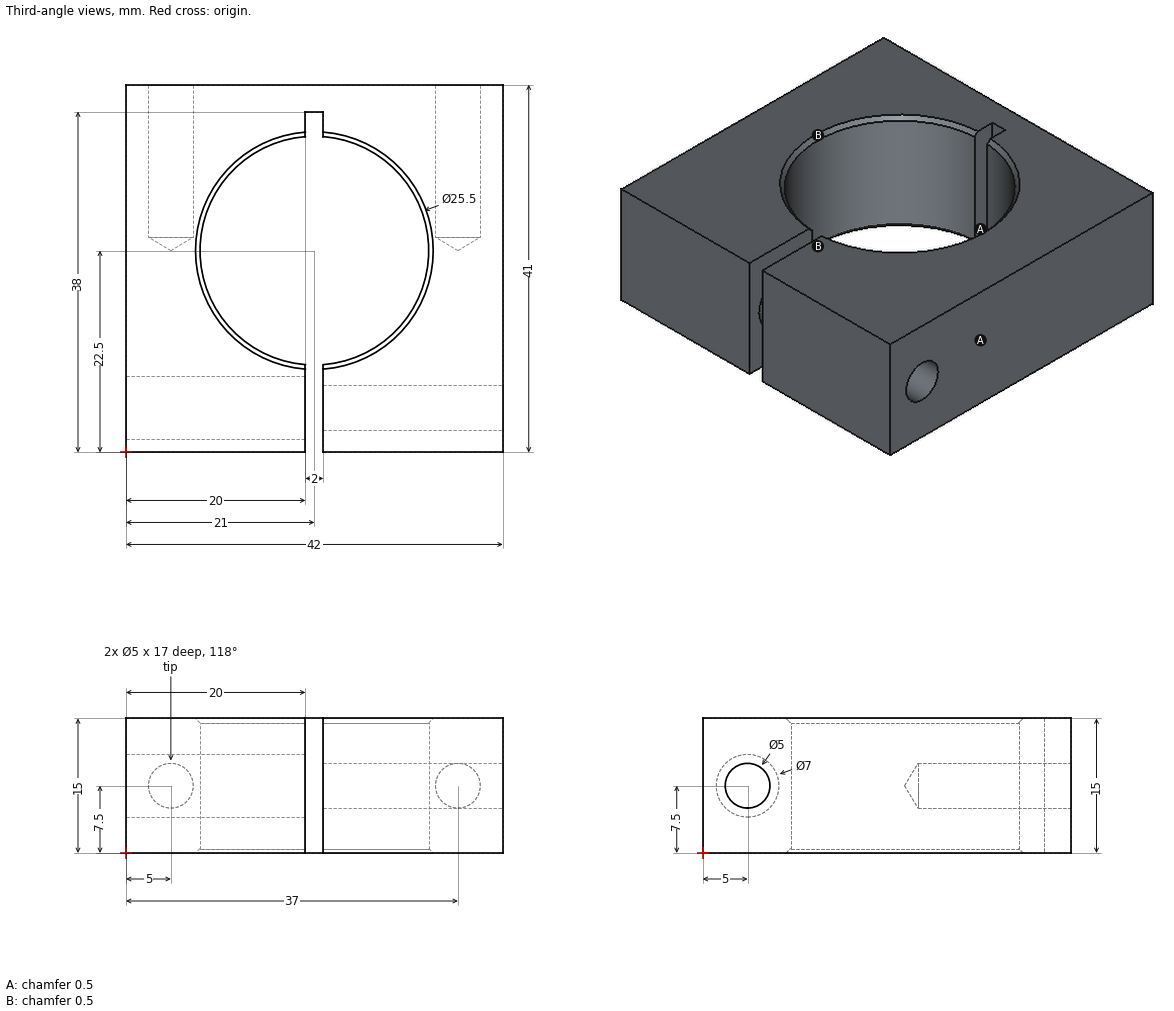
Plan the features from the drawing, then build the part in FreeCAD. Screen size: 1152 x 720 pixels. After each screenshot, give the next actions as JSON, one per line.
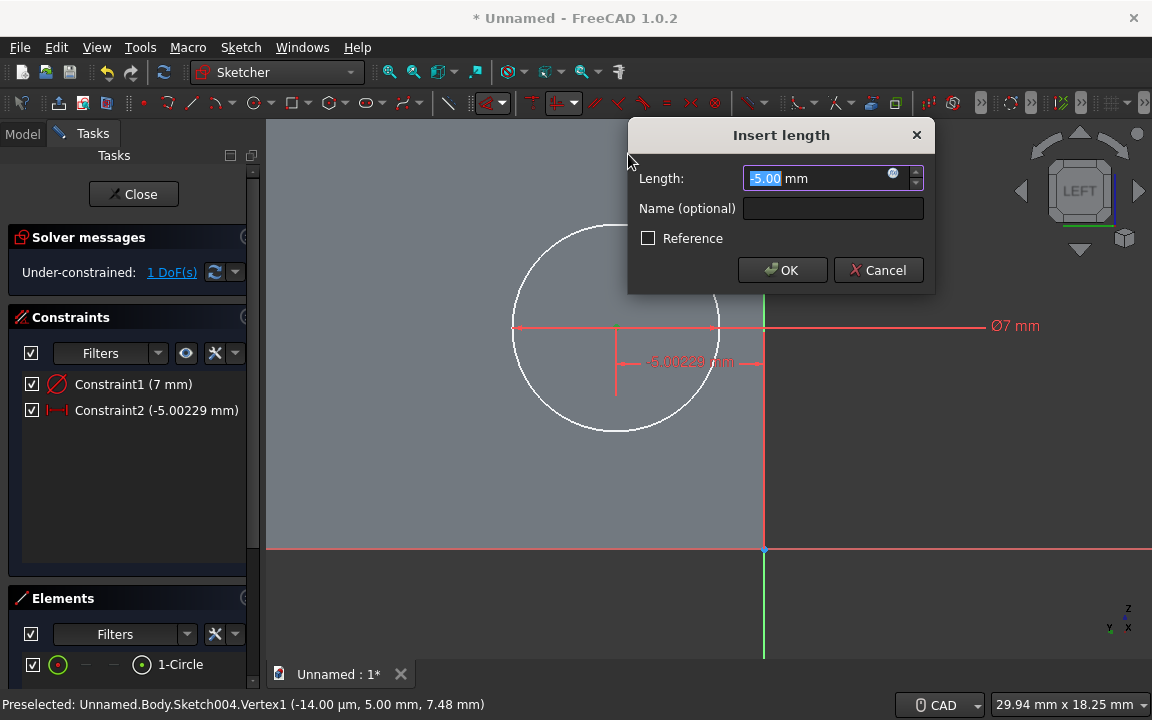
{"action": "type", "text": "-5"}
{"action": "key", "text": "Return"}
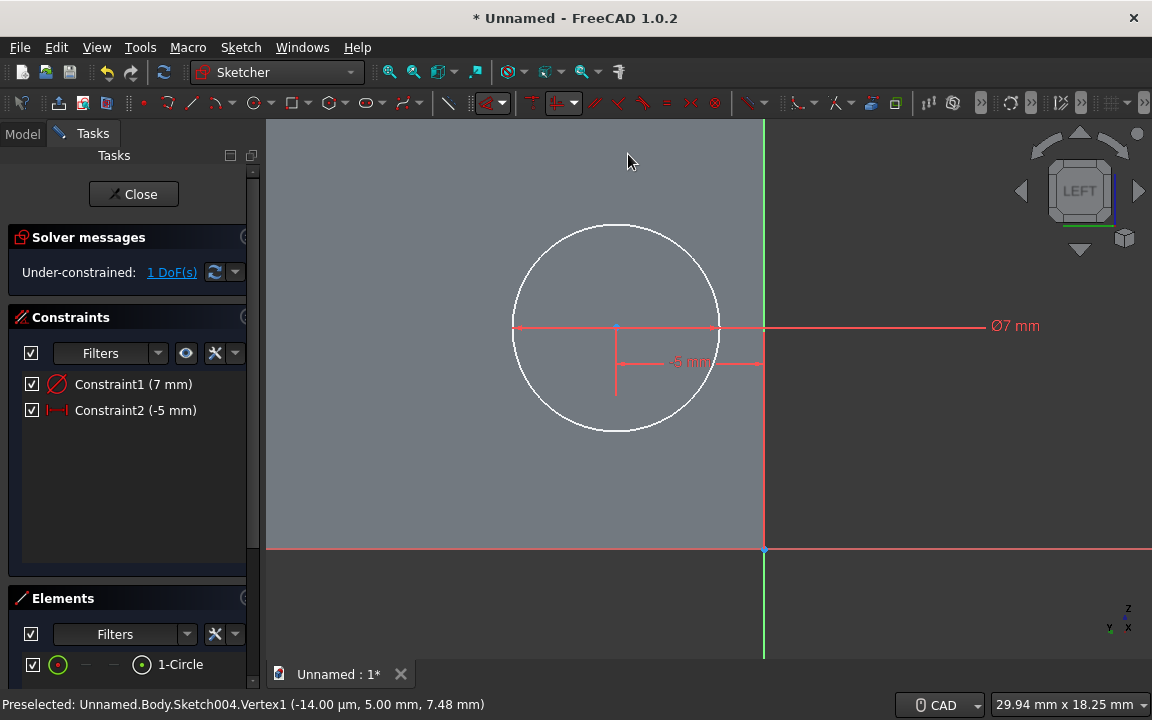
{"action": "left_click", "coordinate": [616, 328]}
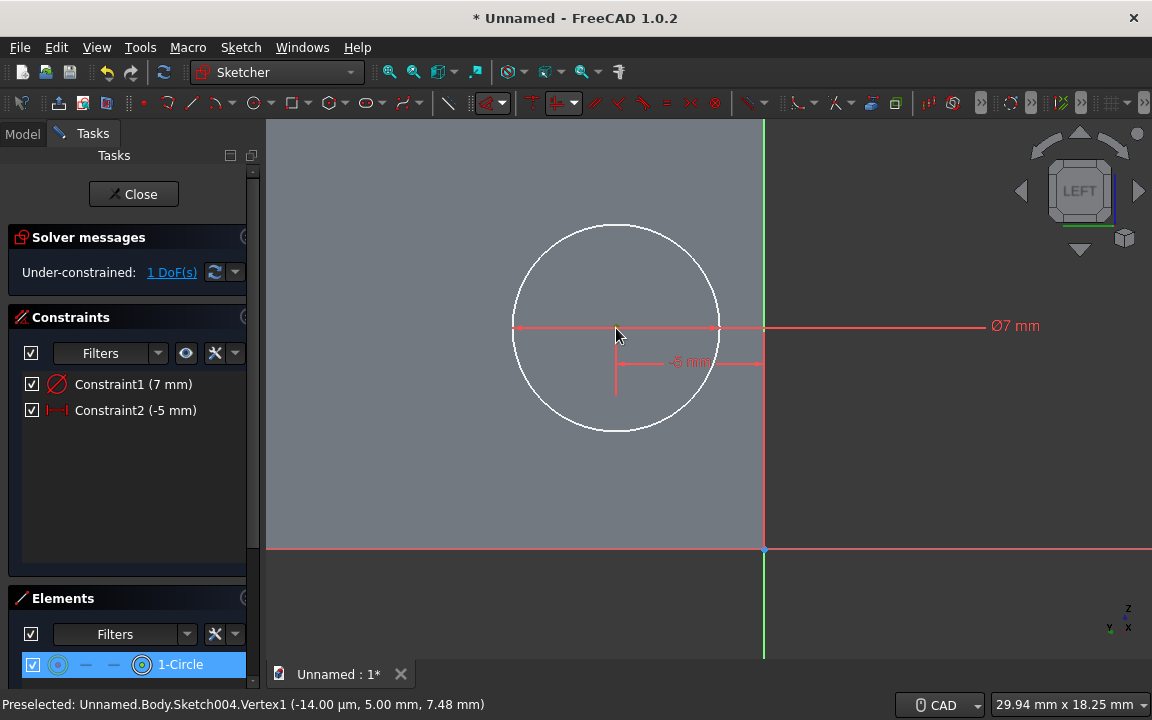
{"action": "left_click", "coordinate": [504, 104]}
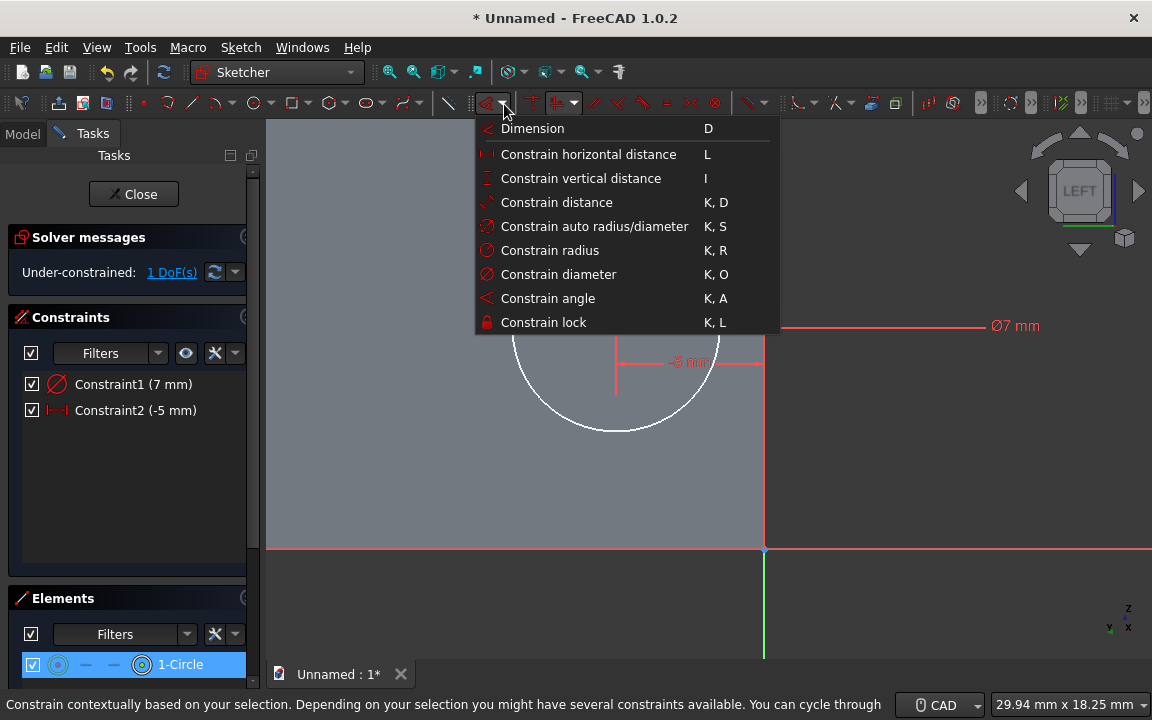
{"action": "left_click", "coordinate": [628, 178]}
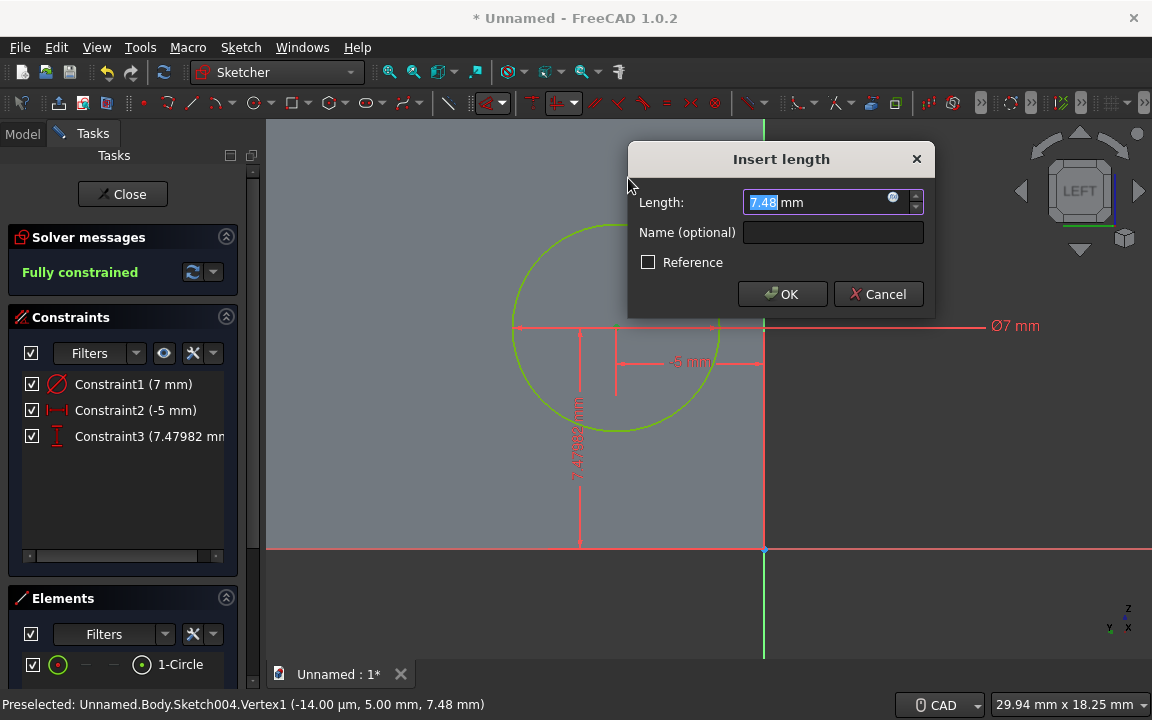
{"action": "type", "text": "7.5"}
{"action": "key", "text": "Return"}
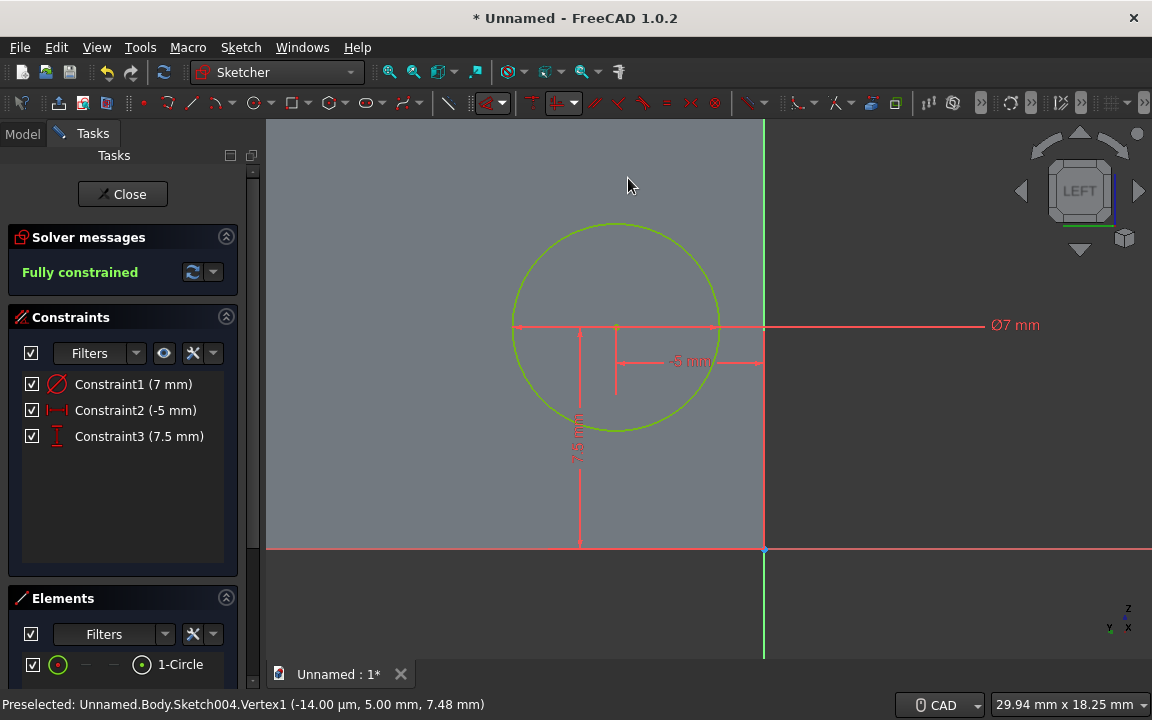
{"action": "left_click", "coordinate": [123, 194]}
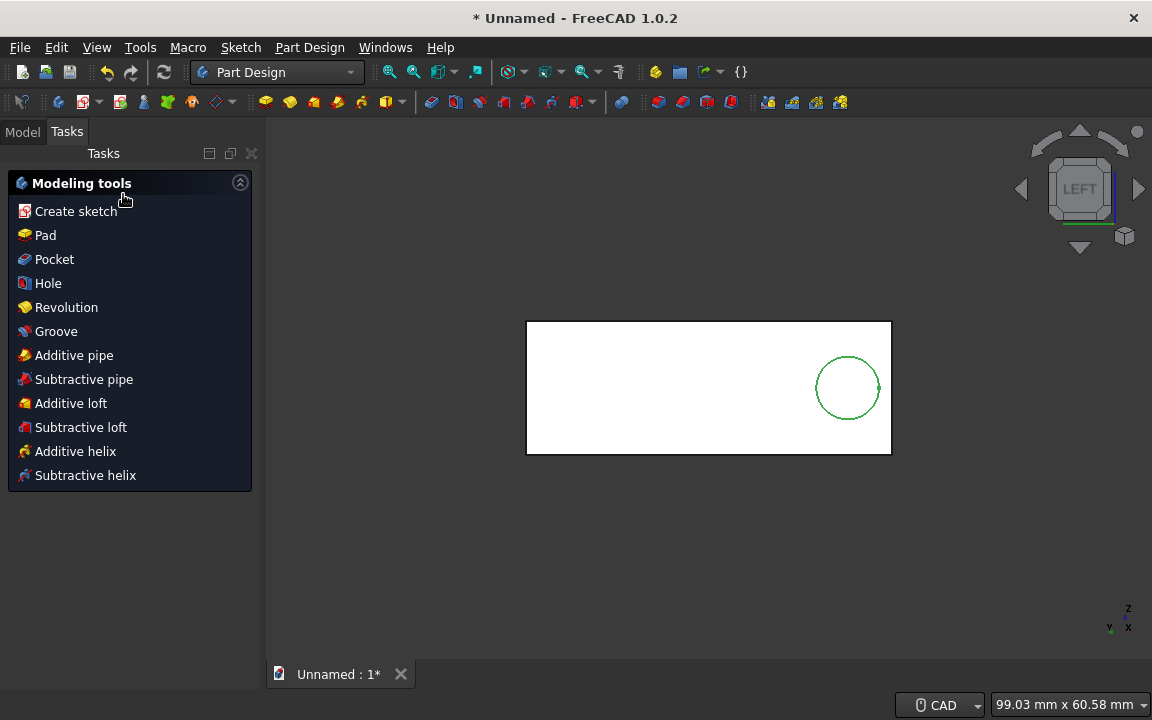
{"action": "left_click", "coordinate": [432, 102]}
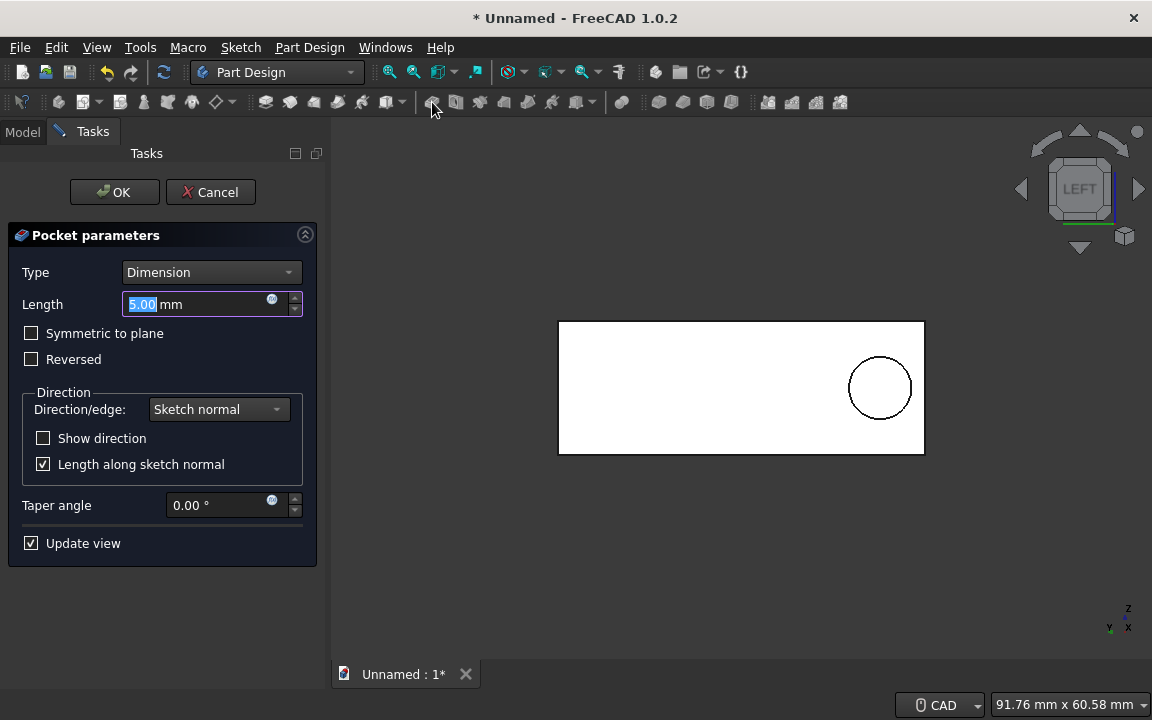
{"action": "type", "text": "20"}
{"action": "key", "text": "Tab"}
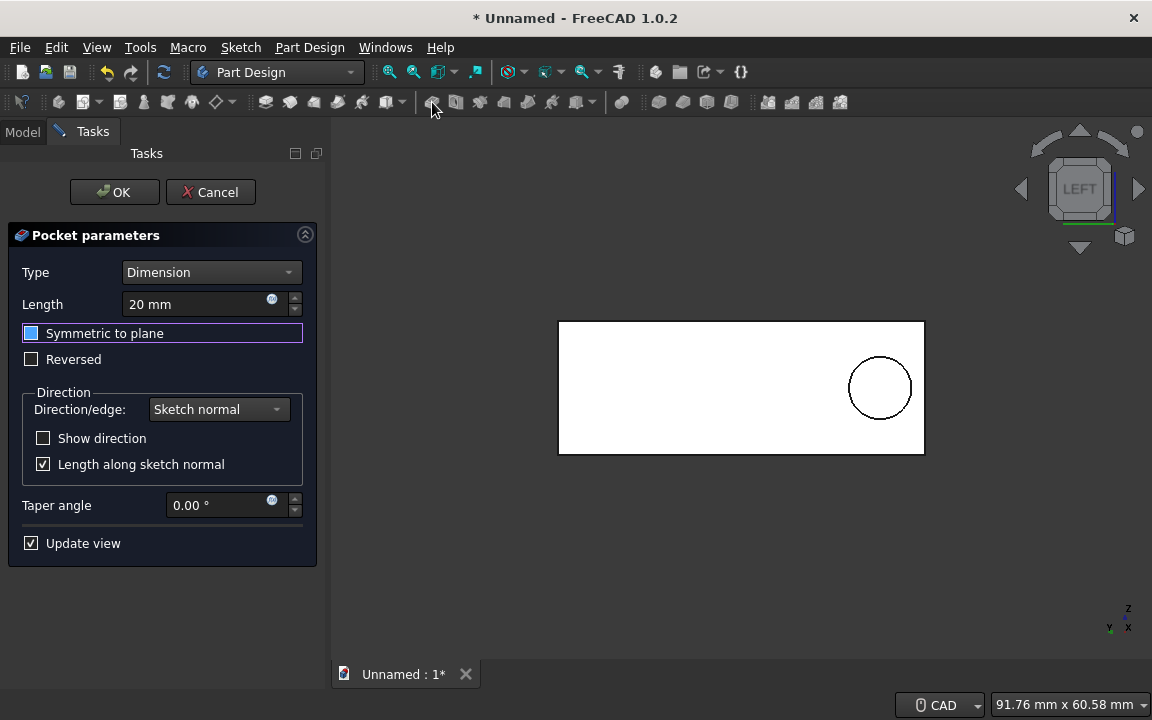
{"action": "left_click", "coordinate": [115, 192]}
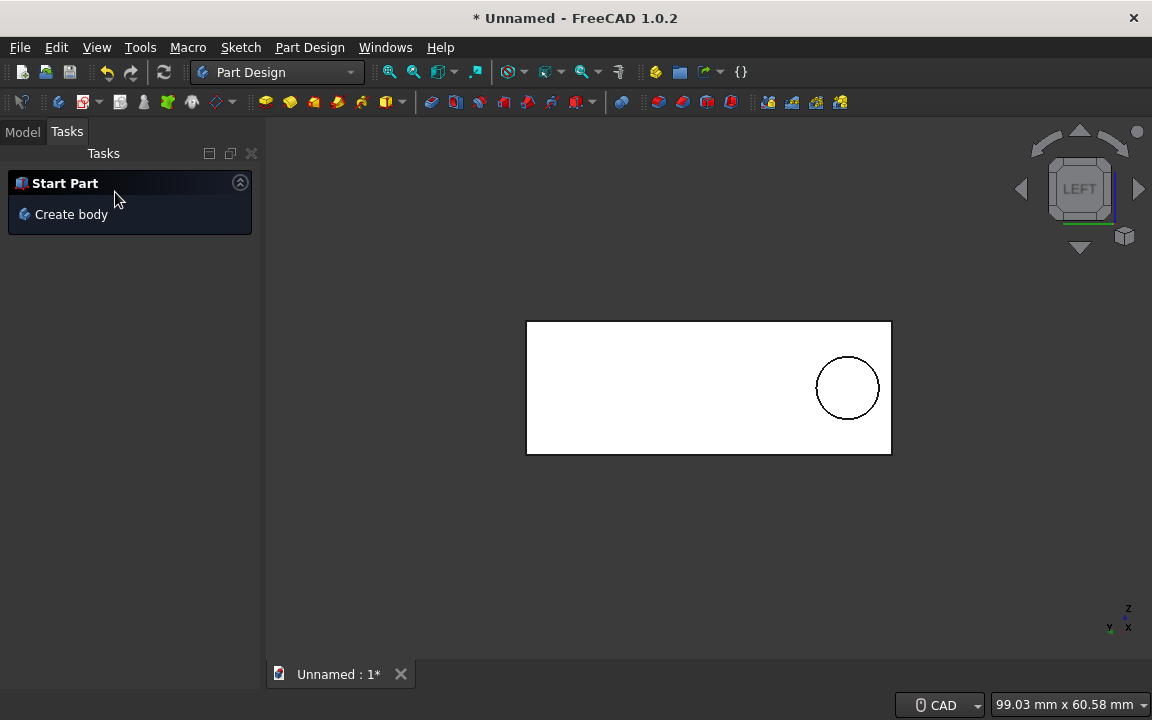
{"action": "left_click", "coordinate": [390, 72]}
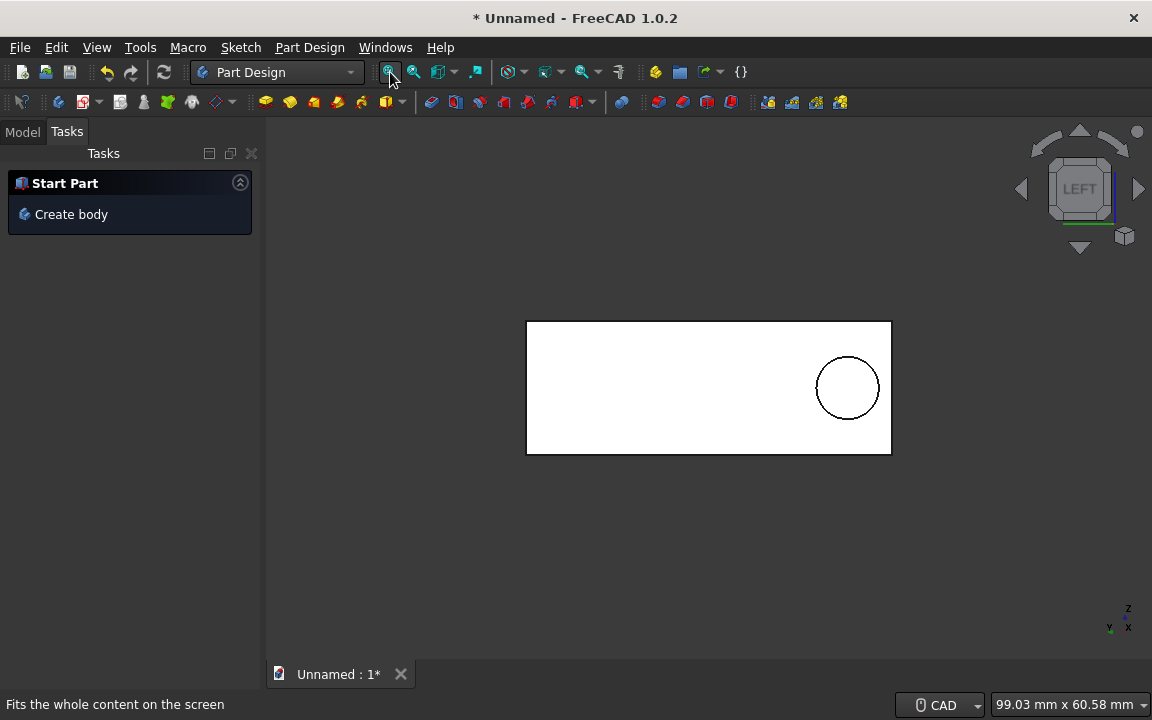
{"action": "left_click", "coordinate": [849, 368]}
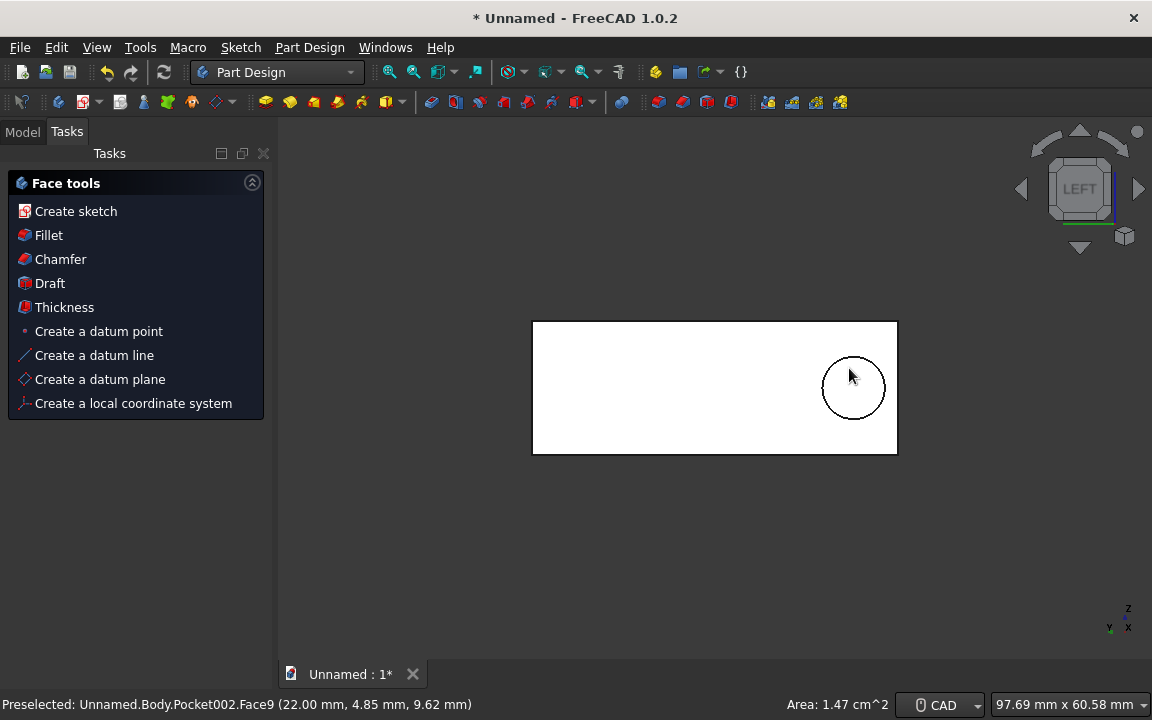
{"action": "left_click", "coordinate": [84, 102]}